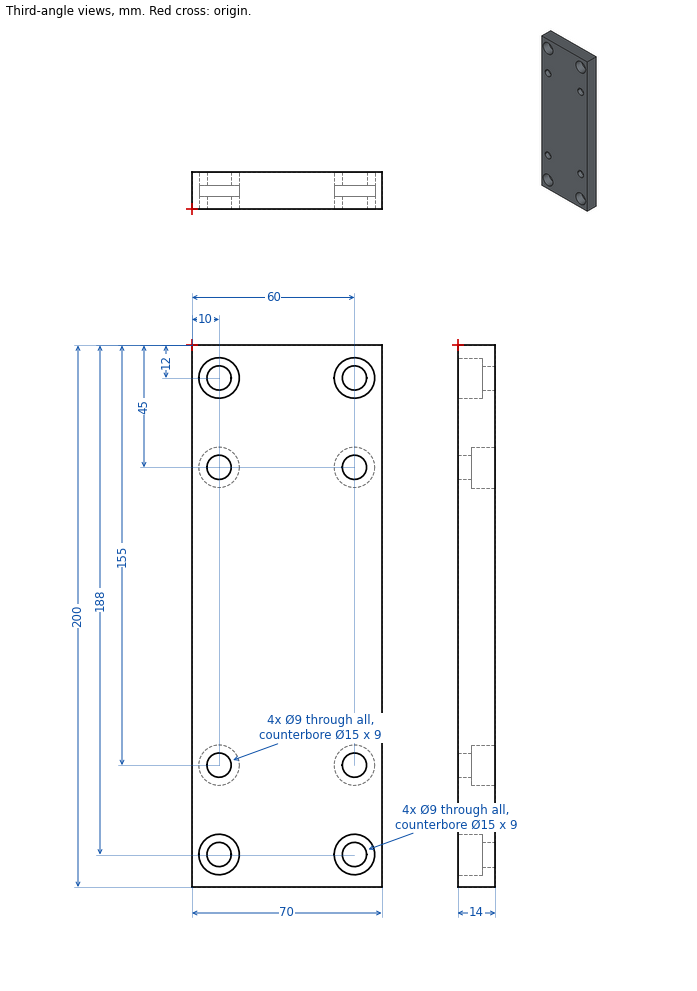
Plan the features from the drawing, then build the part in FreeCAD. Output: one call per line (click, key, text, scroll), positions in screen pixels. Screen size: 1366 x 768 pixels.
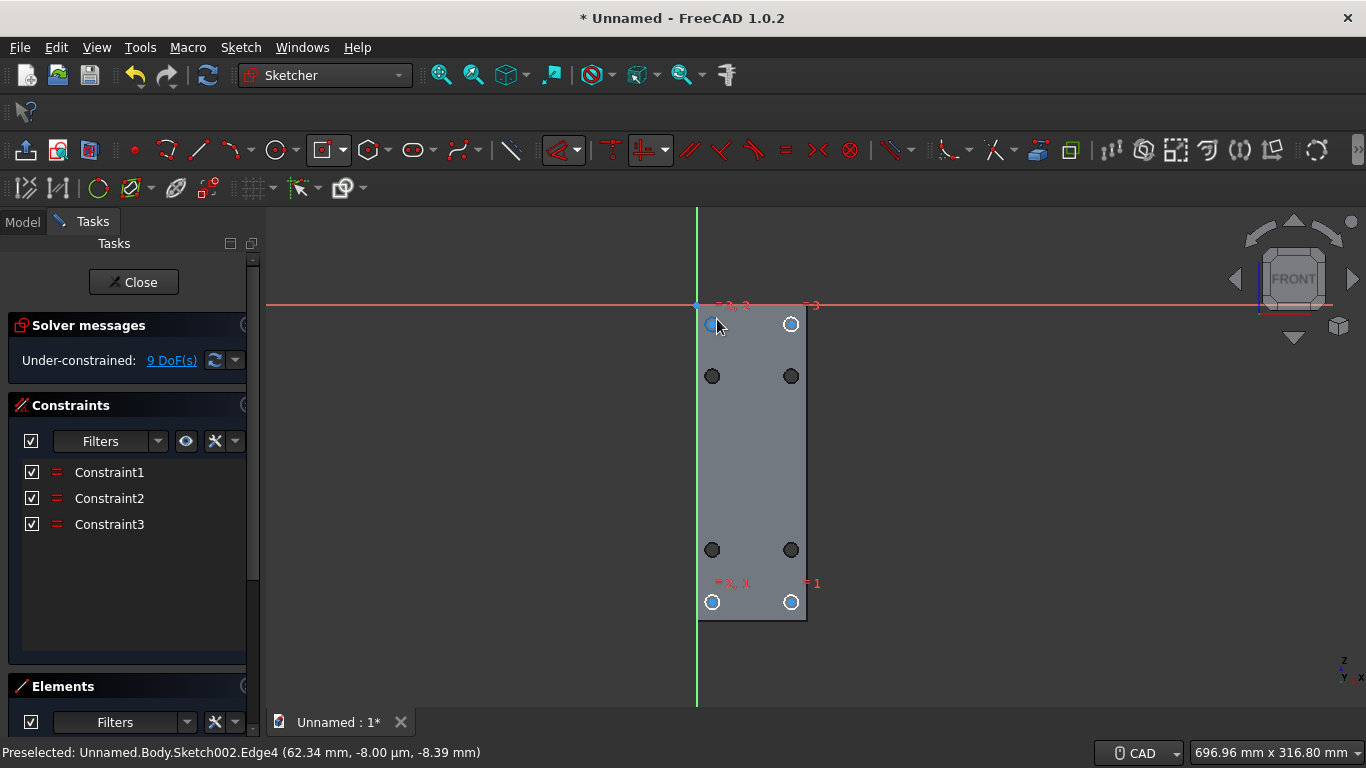
click(791, 602)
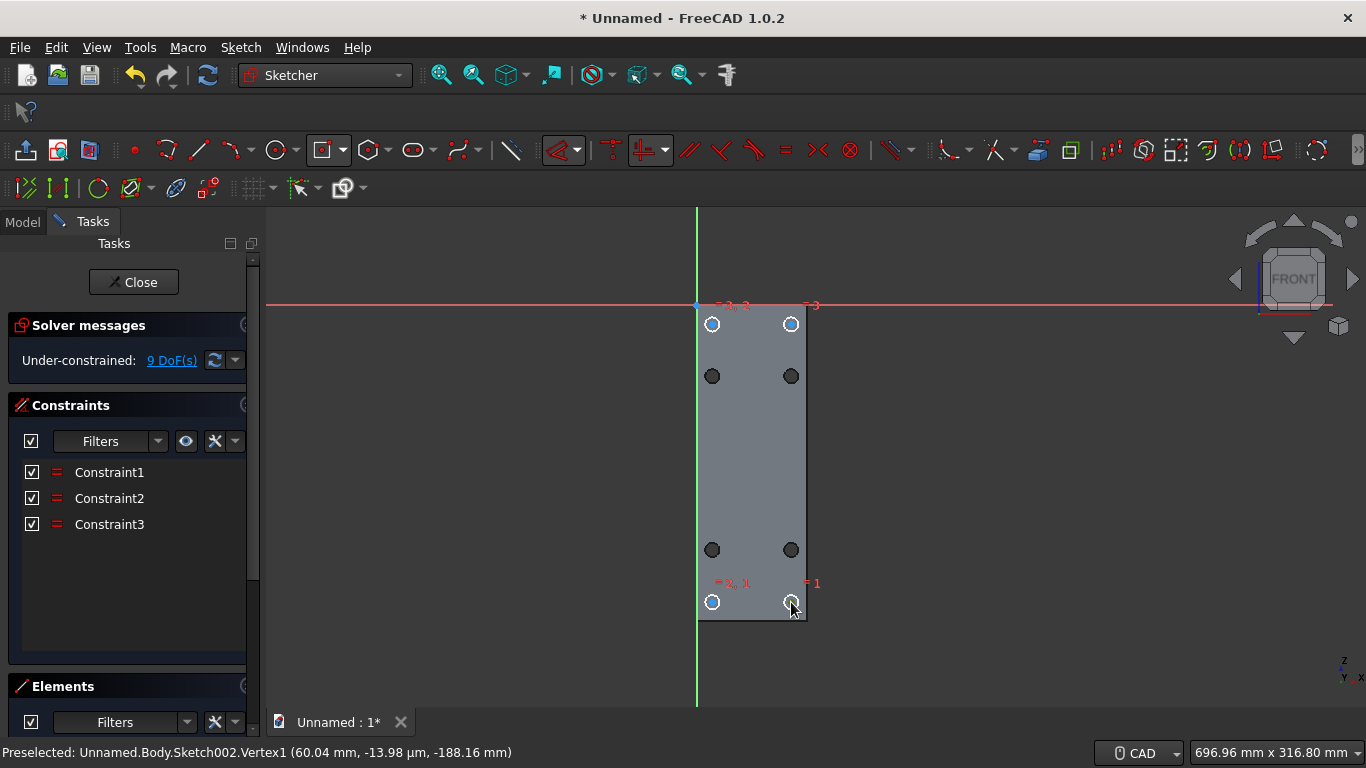
click(712, 602)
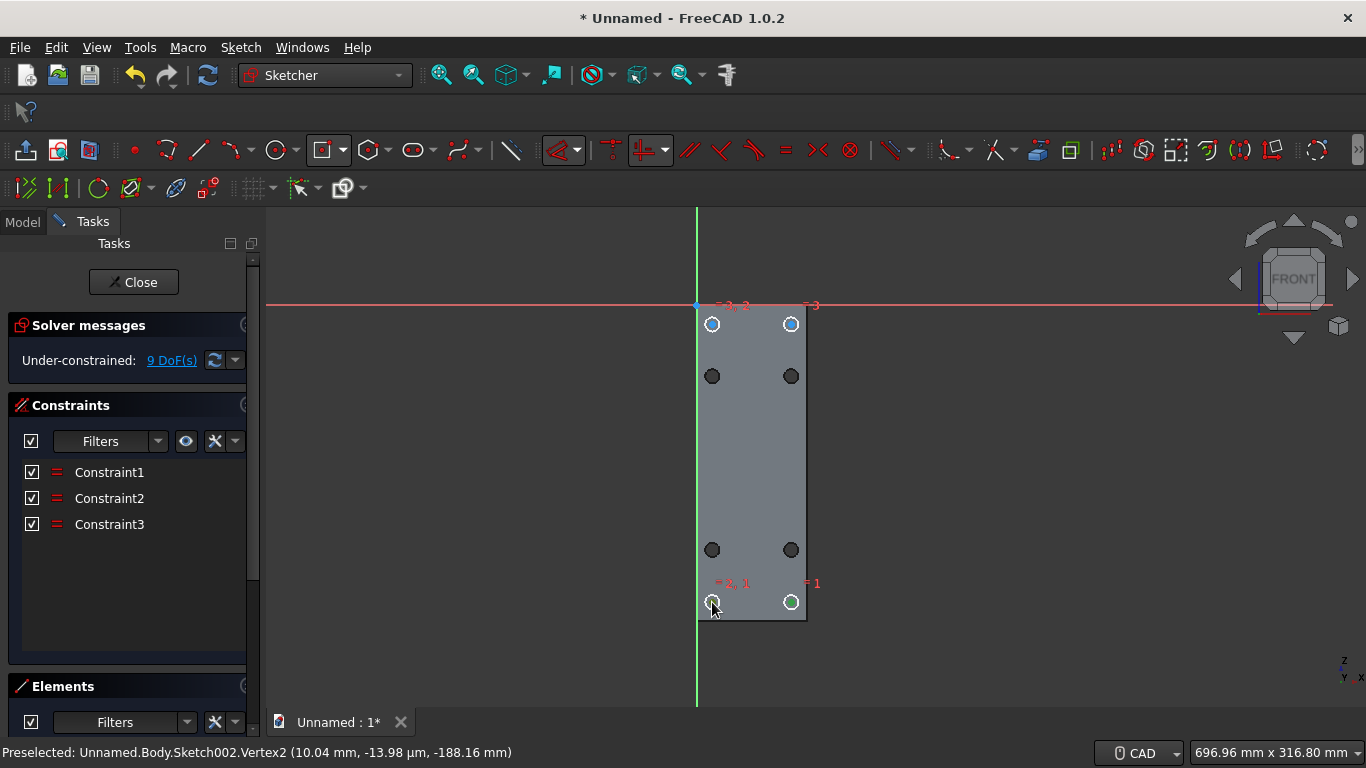
key(h)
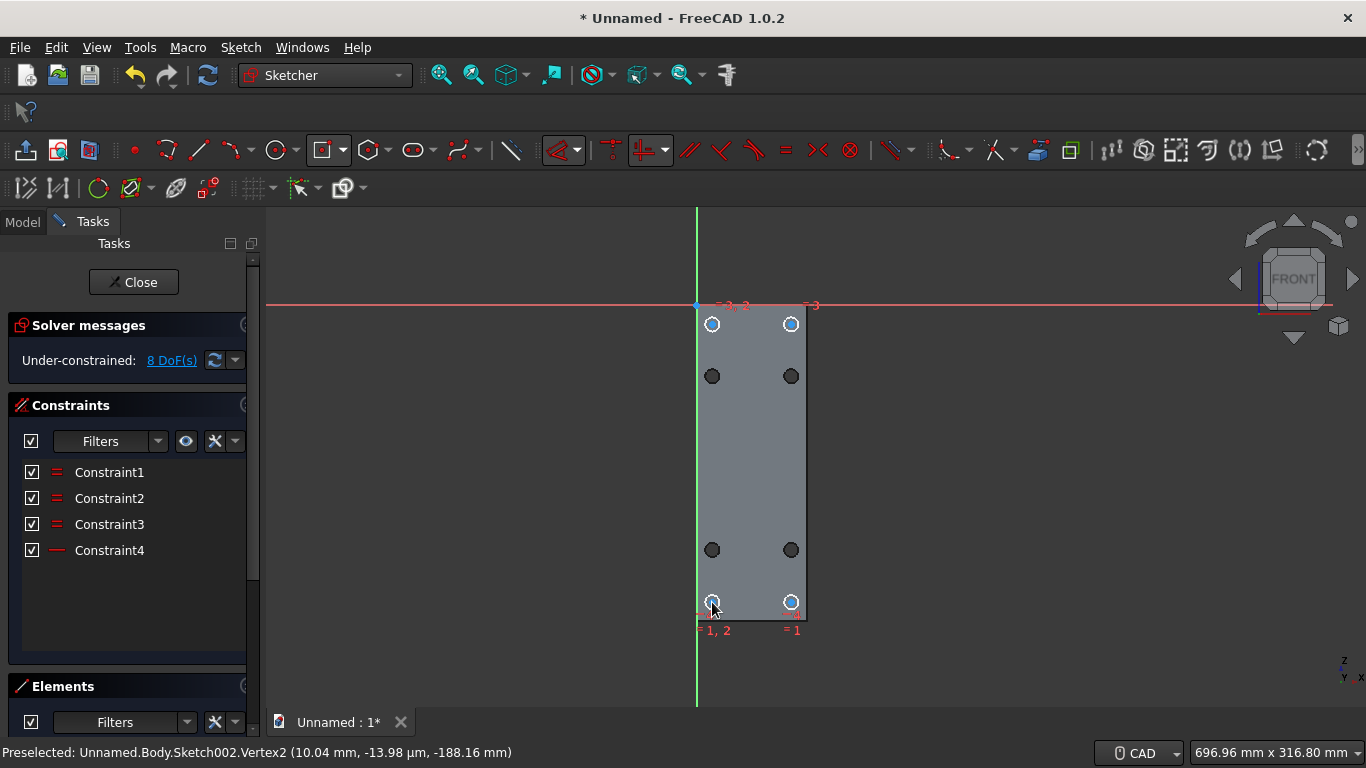
click(712, 602)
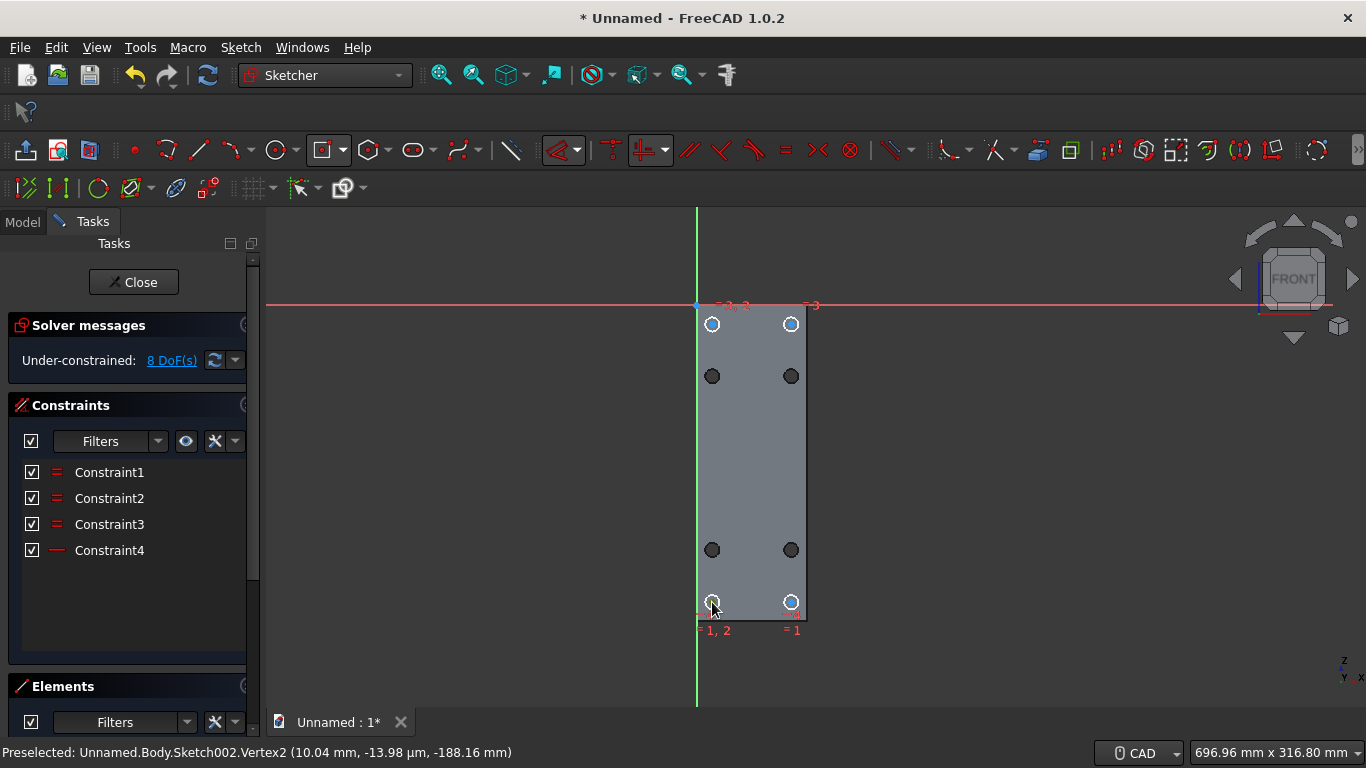
click(712, 324)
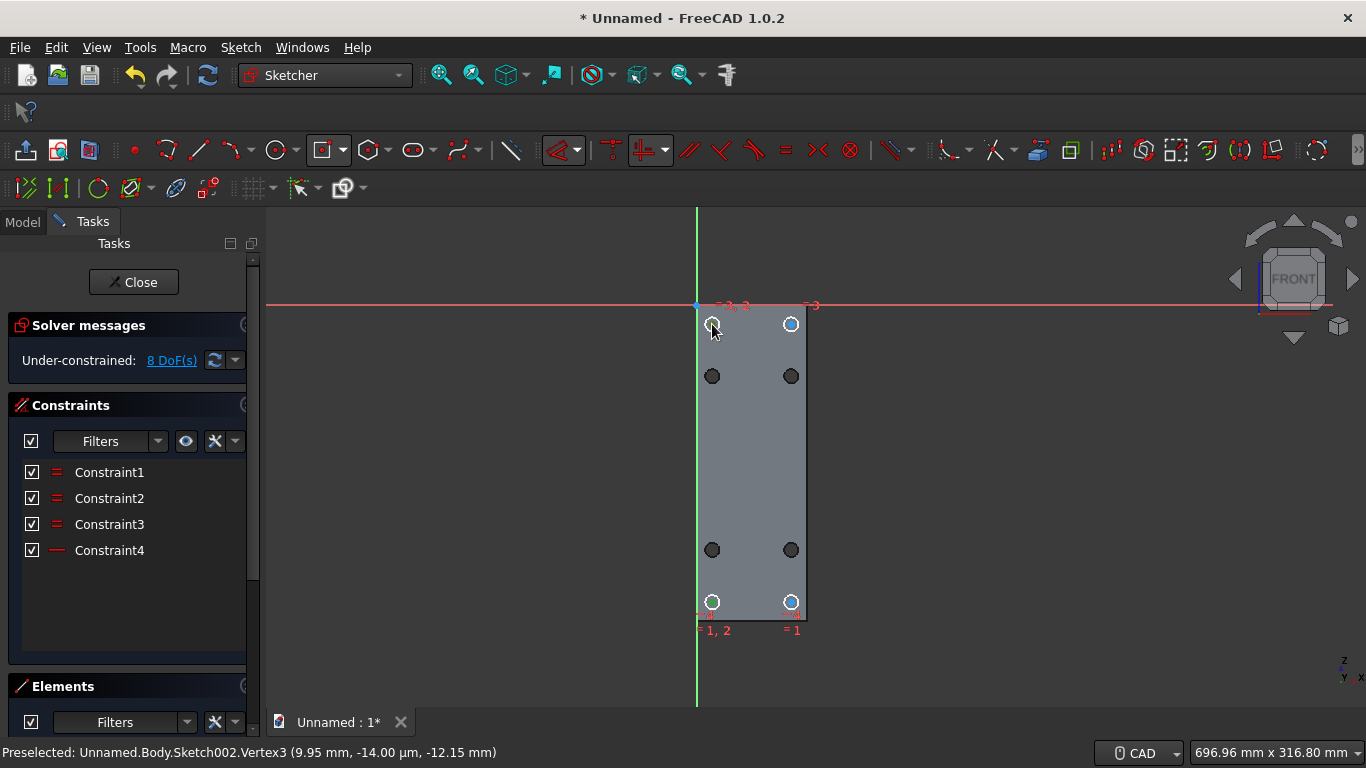
key(v)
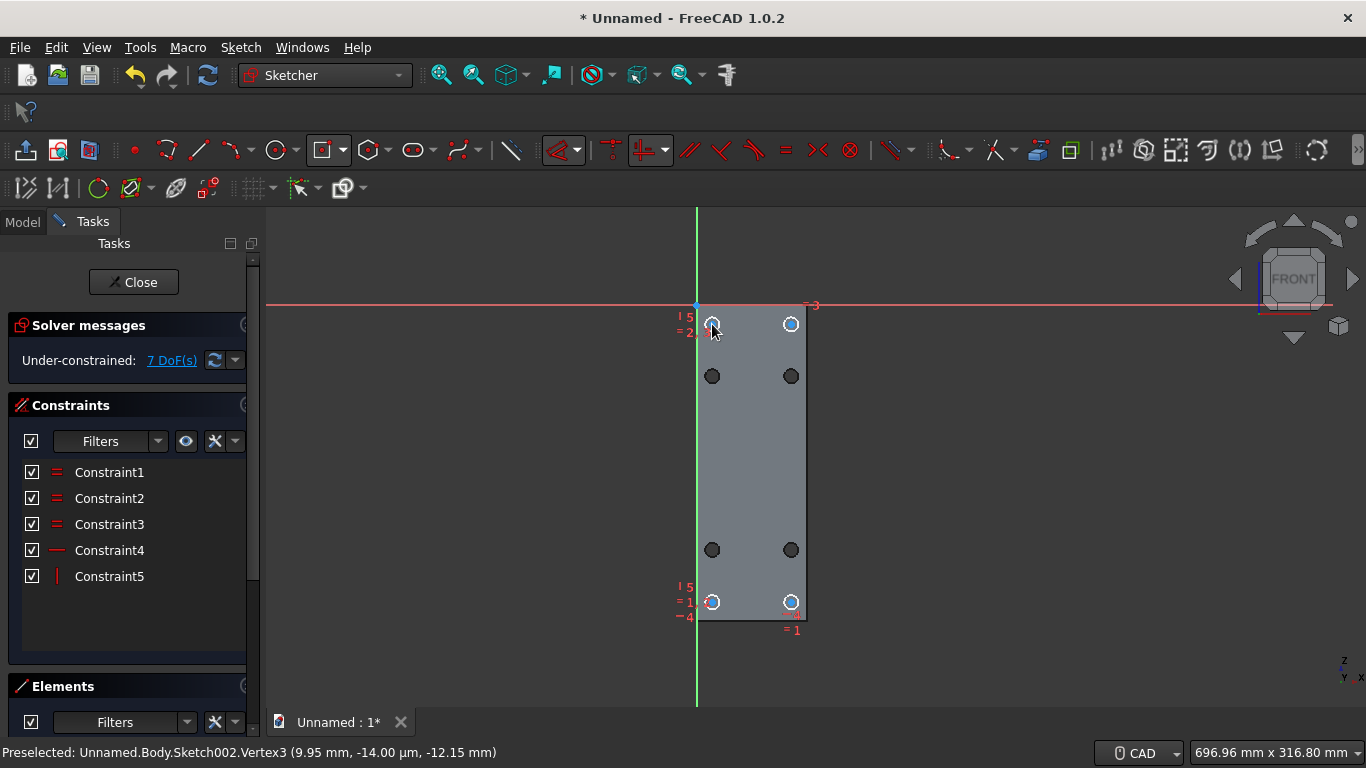
click(791, 602)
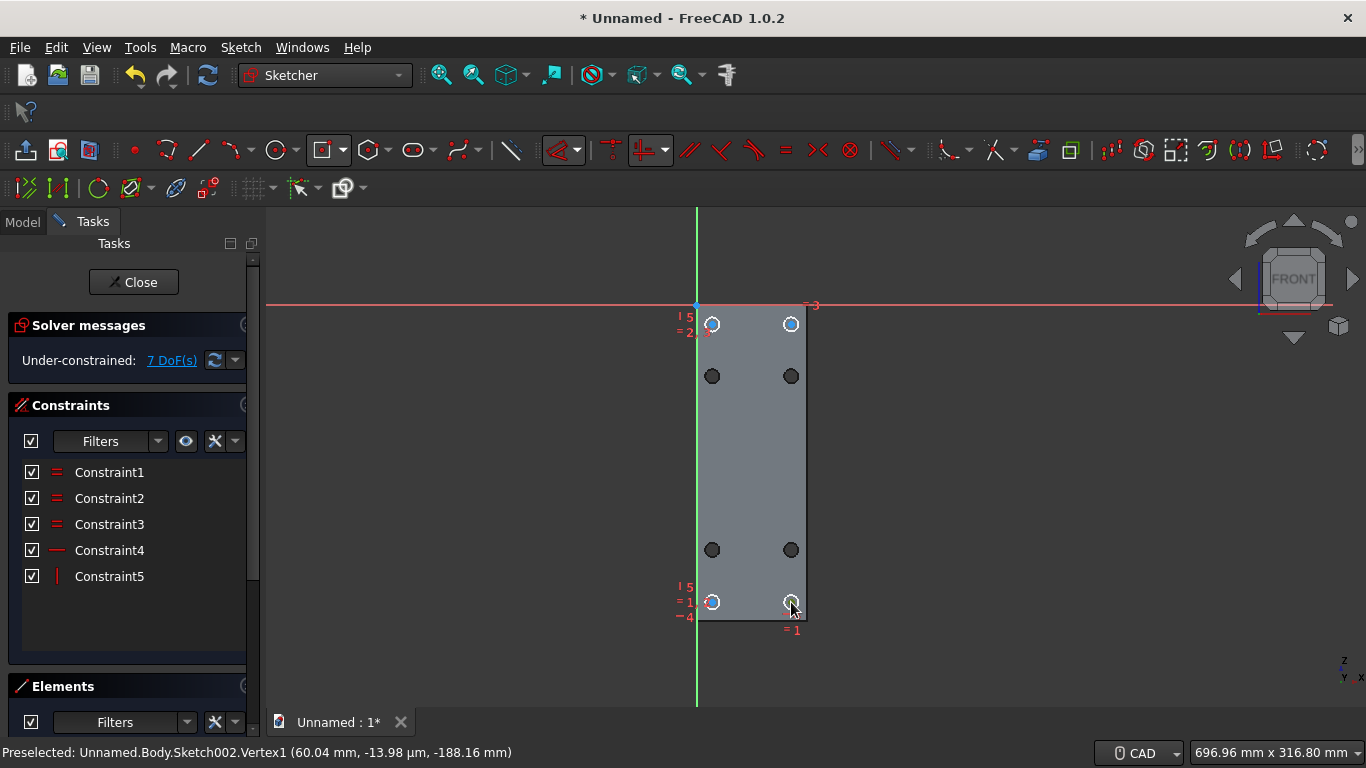
click(791, 324)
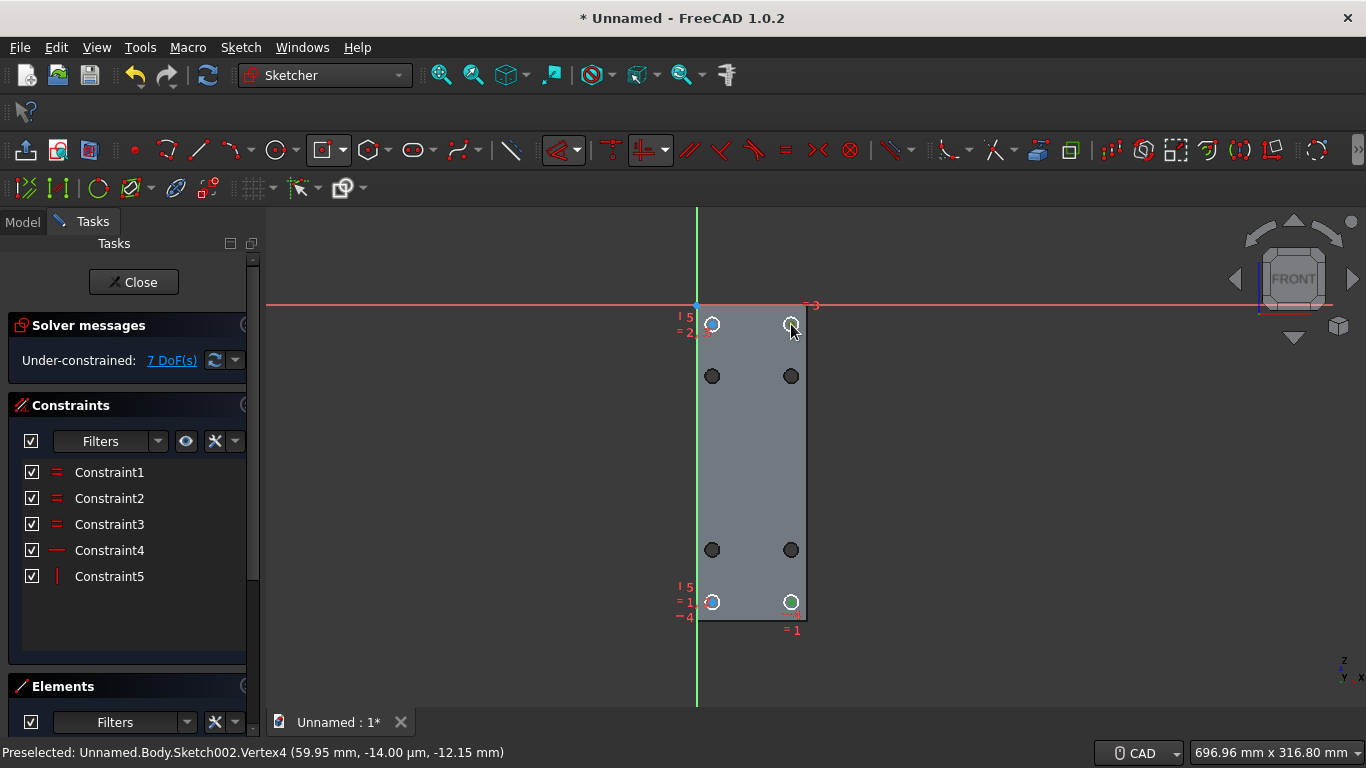
key(v)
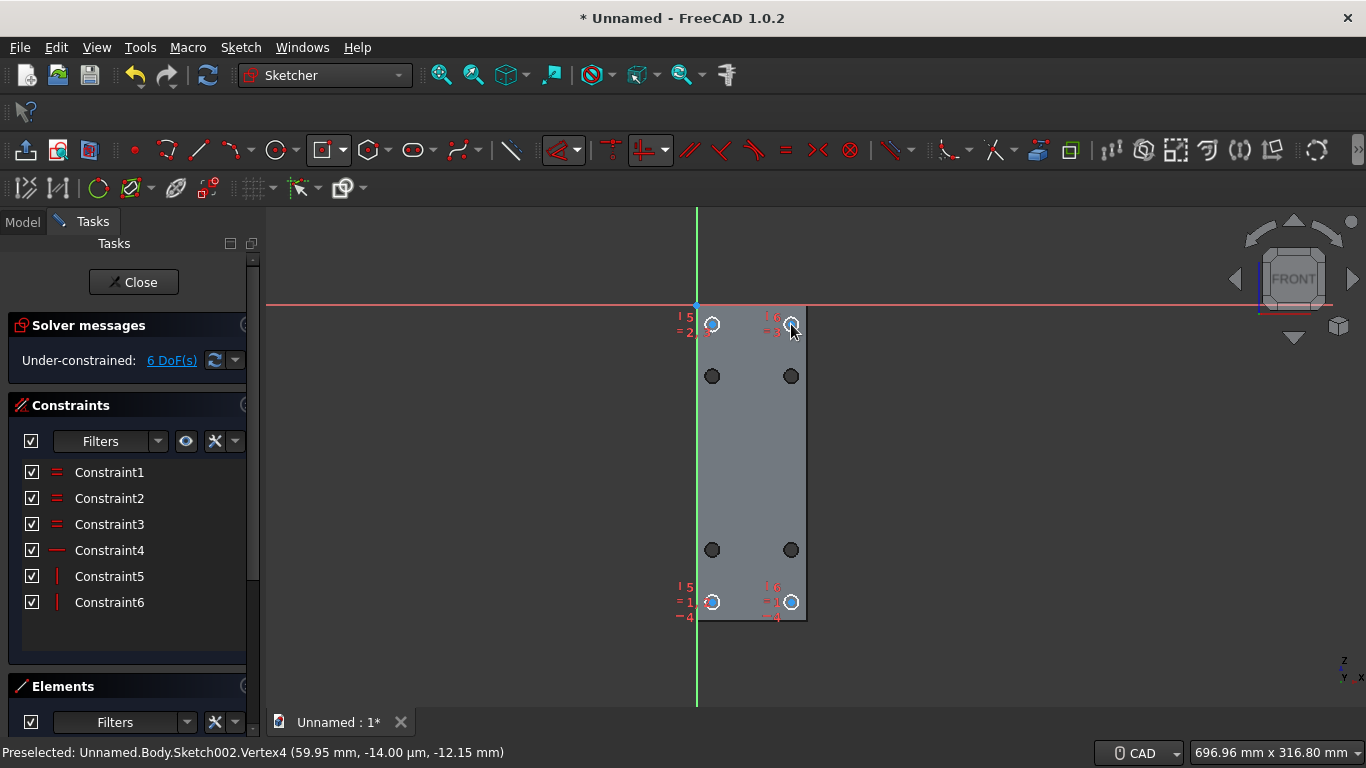
click(712, 324)